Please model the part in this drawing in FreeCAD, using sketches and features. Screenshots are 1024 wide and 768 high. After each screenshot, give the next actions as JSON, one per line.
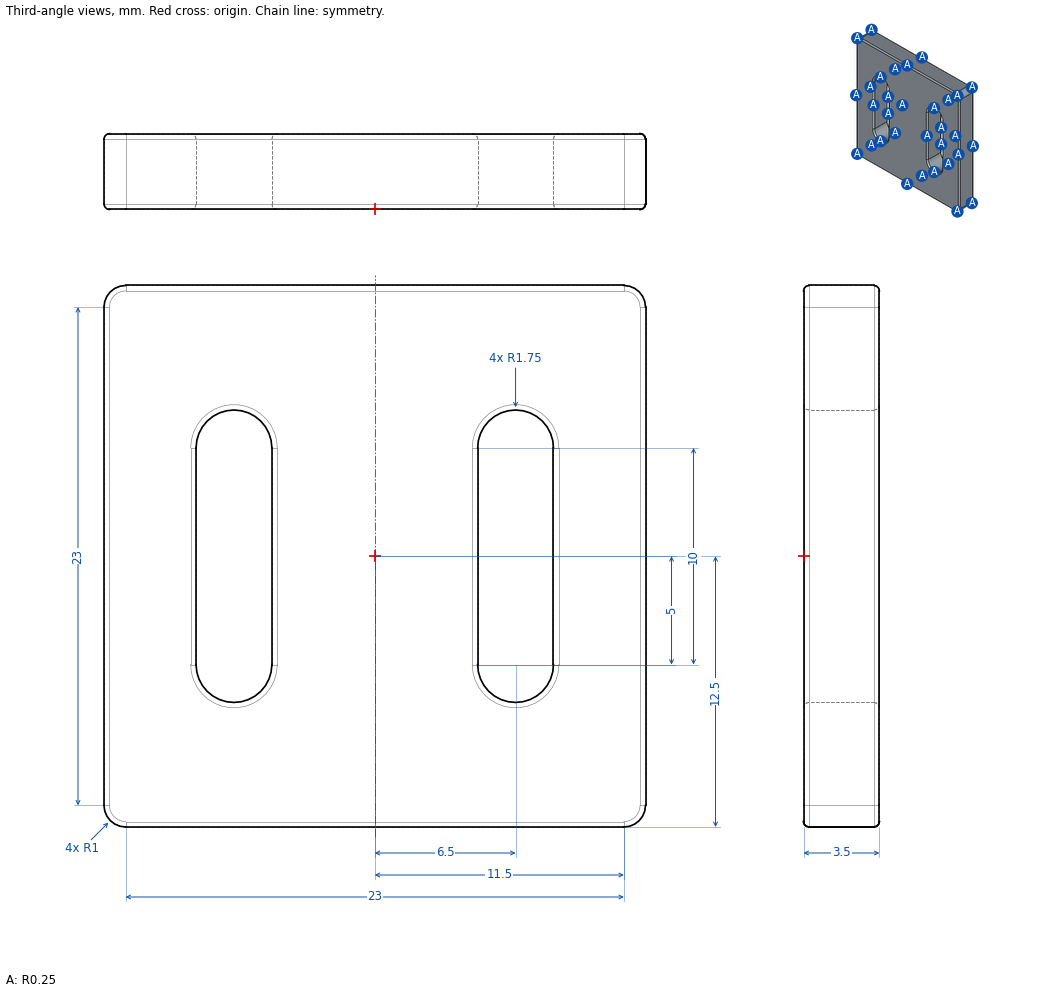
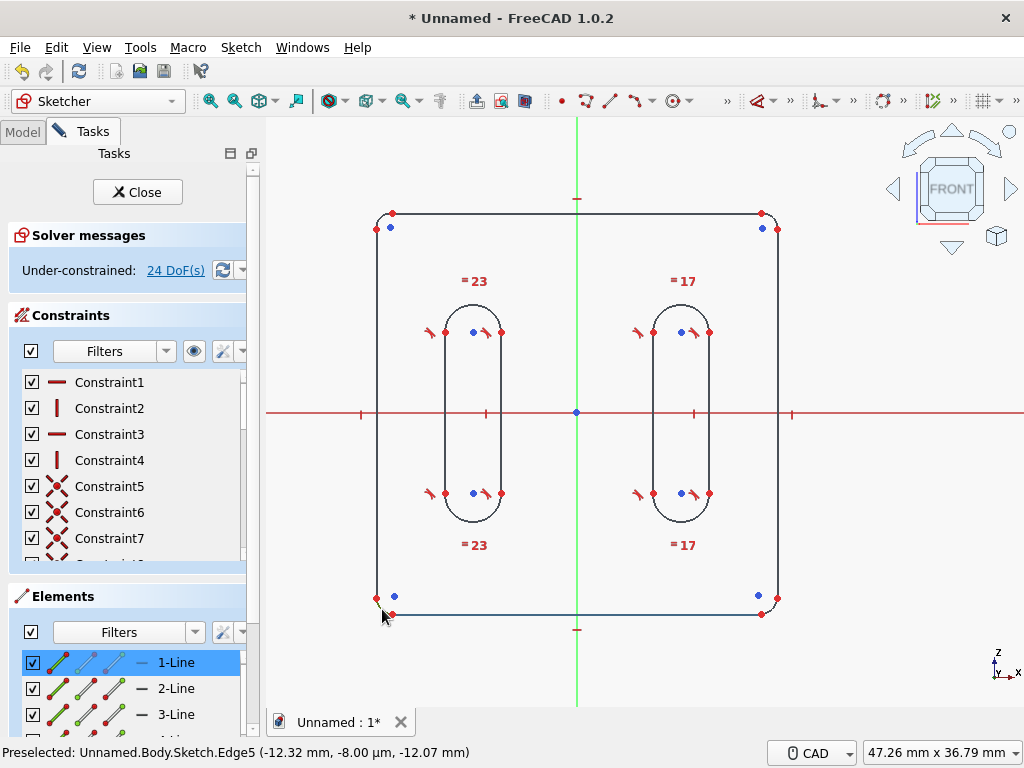
{"action": "key", "text": "t"}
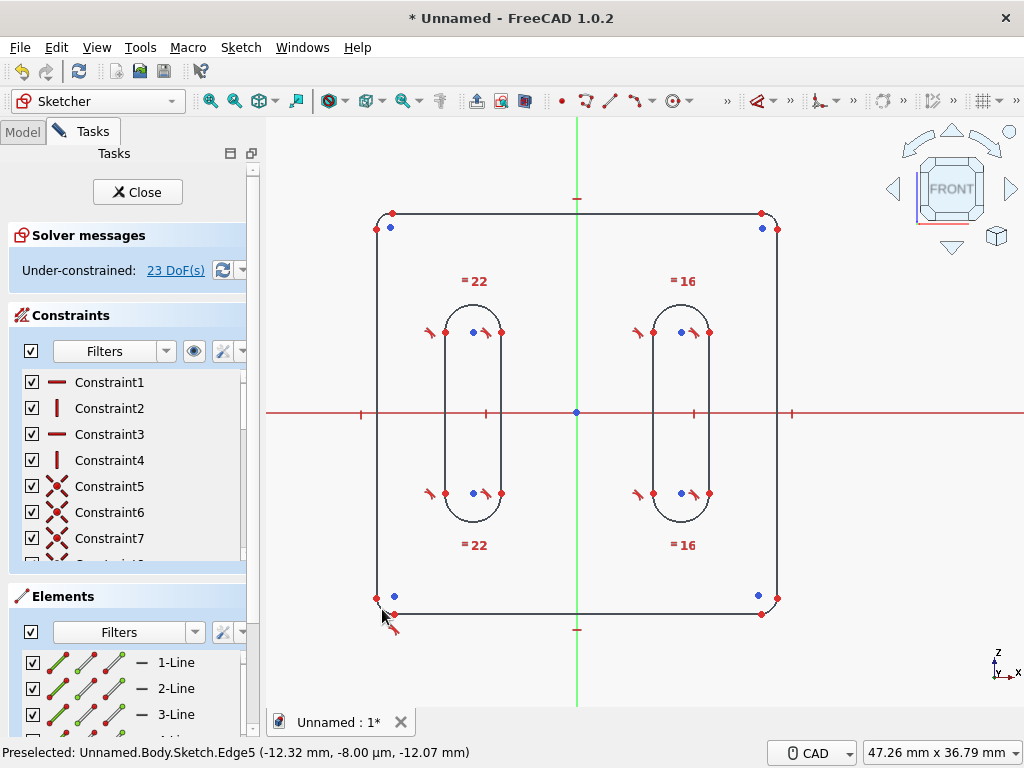
{"action": "left_click", "coordinate": [651, 614]}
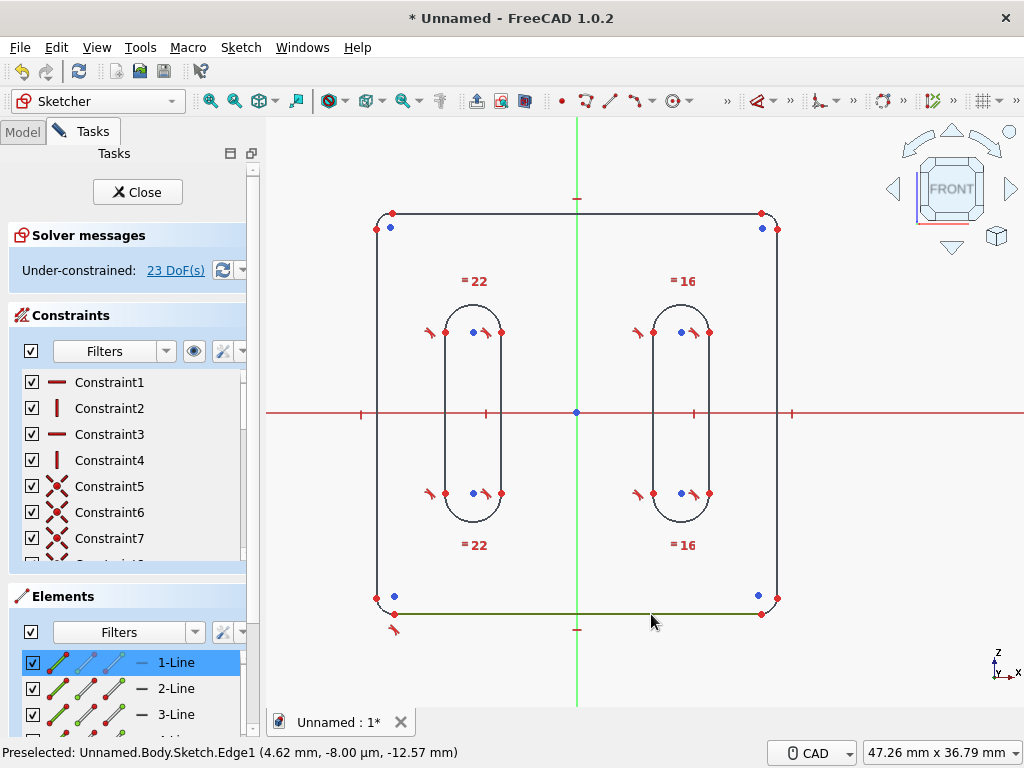
{"action": "left_click", "coordinate": [772, 609]}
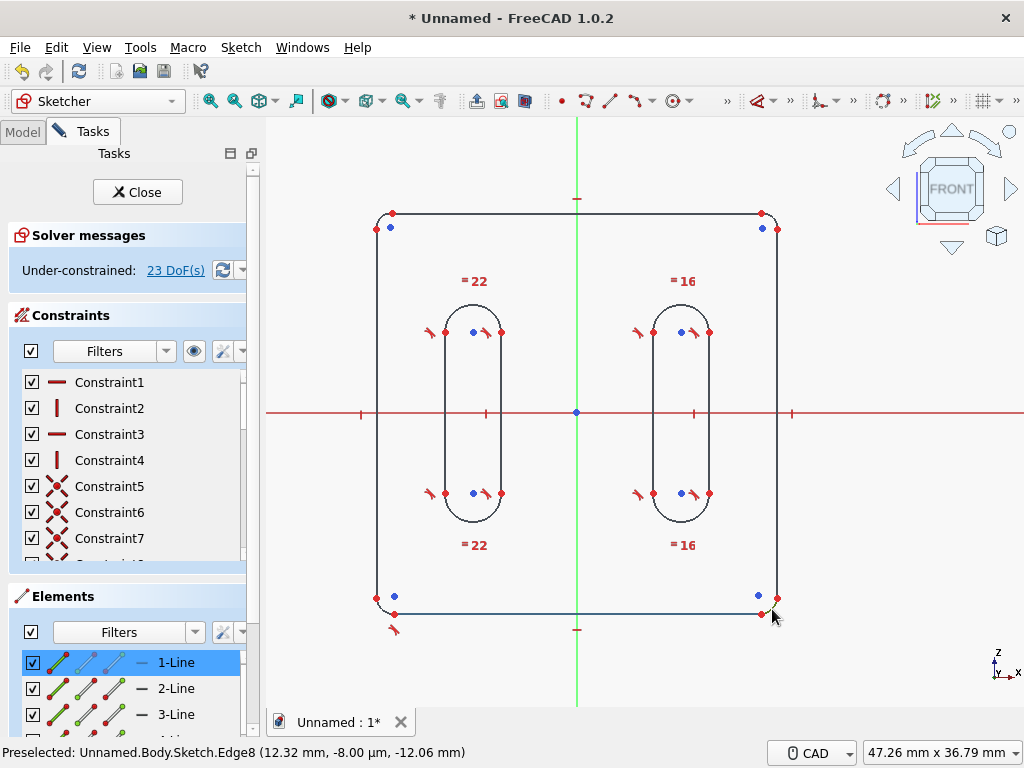
{"action": "key", "text": "t"}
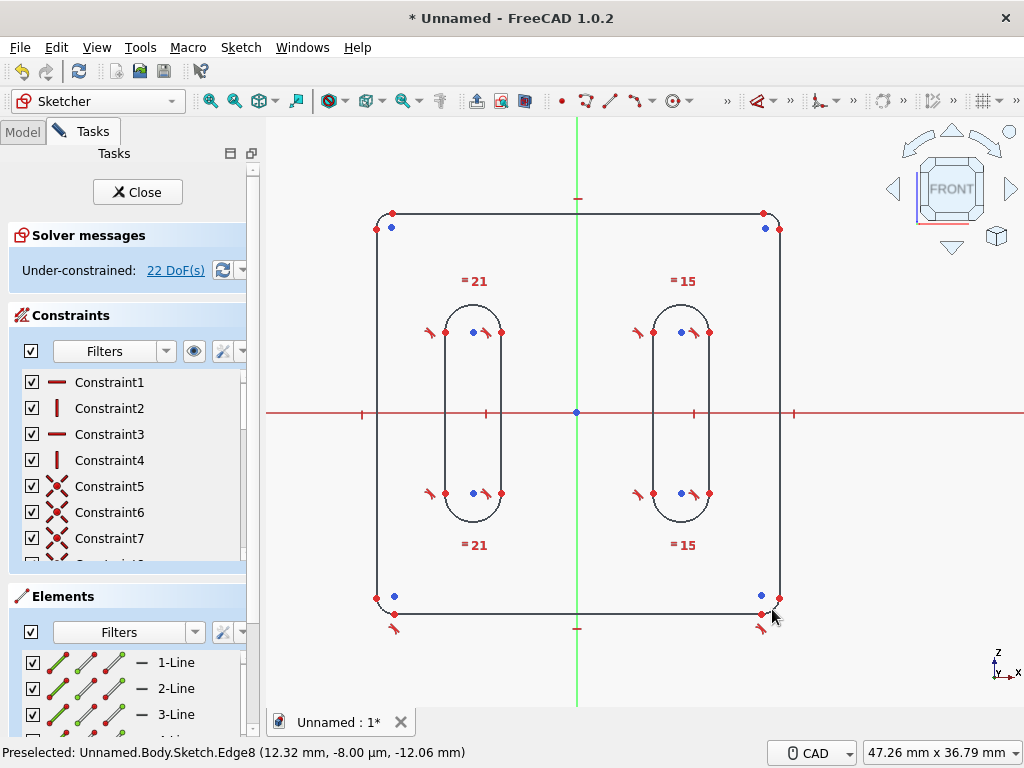
{"action": "left_click", "coordinate": [377, 488]}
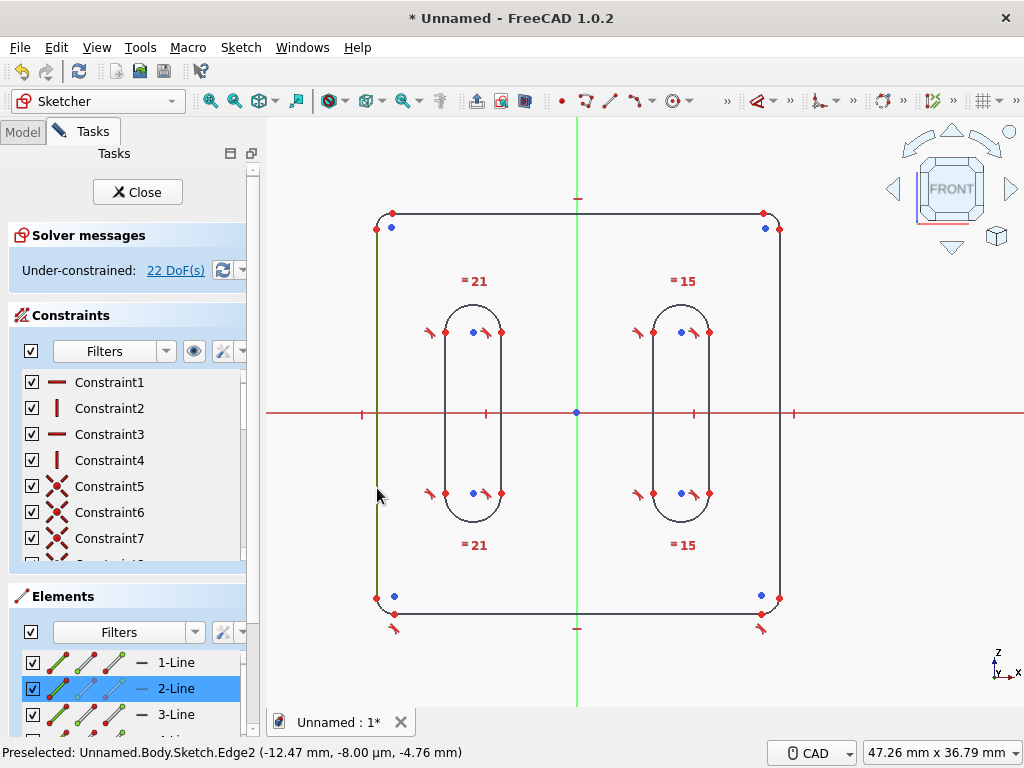
{"action": "left_click", "coordinate": [383, 610]}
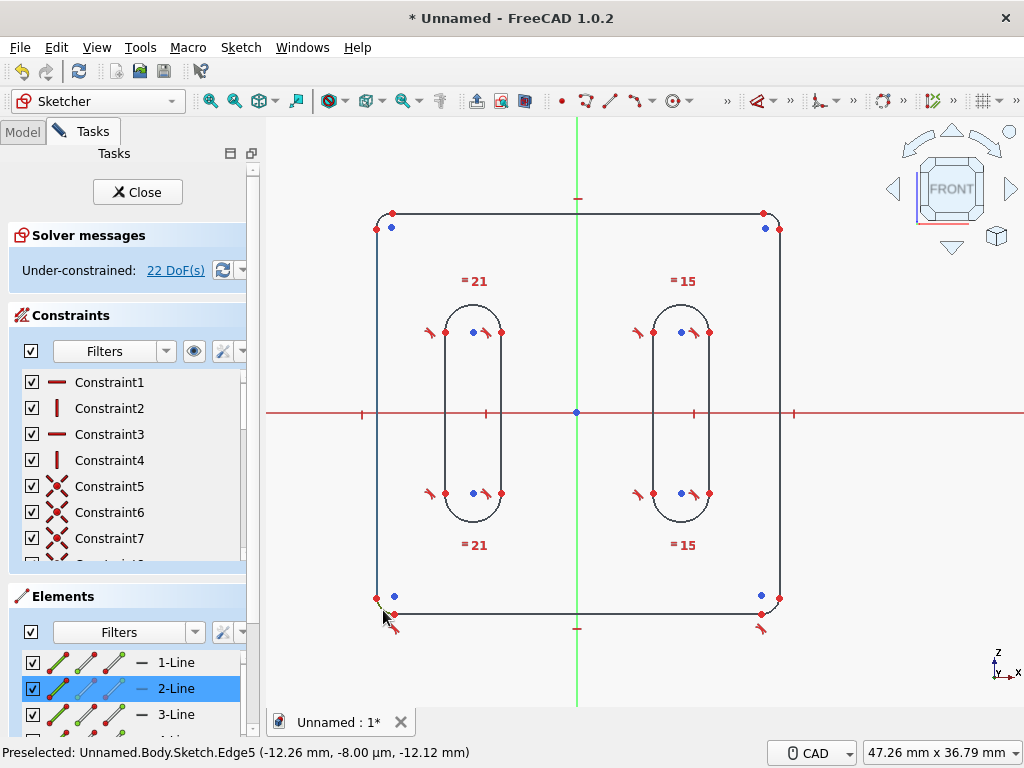
{"action": "key", "text": "t"}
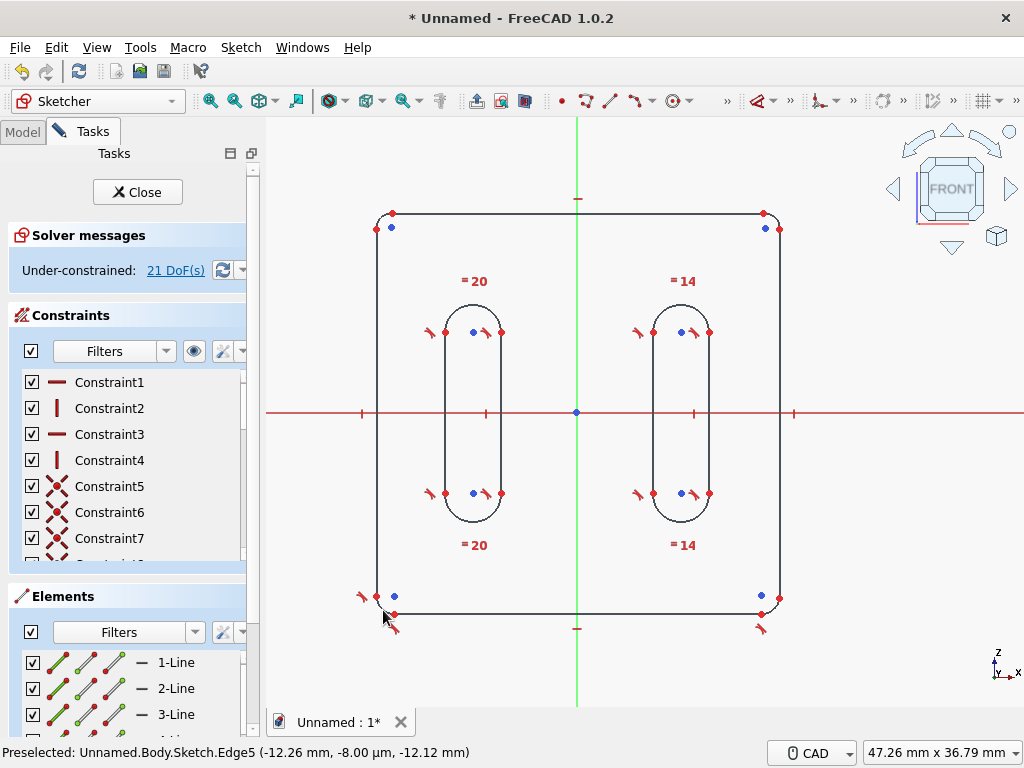
{"action": "left_click", "coordinate": [377, 486]}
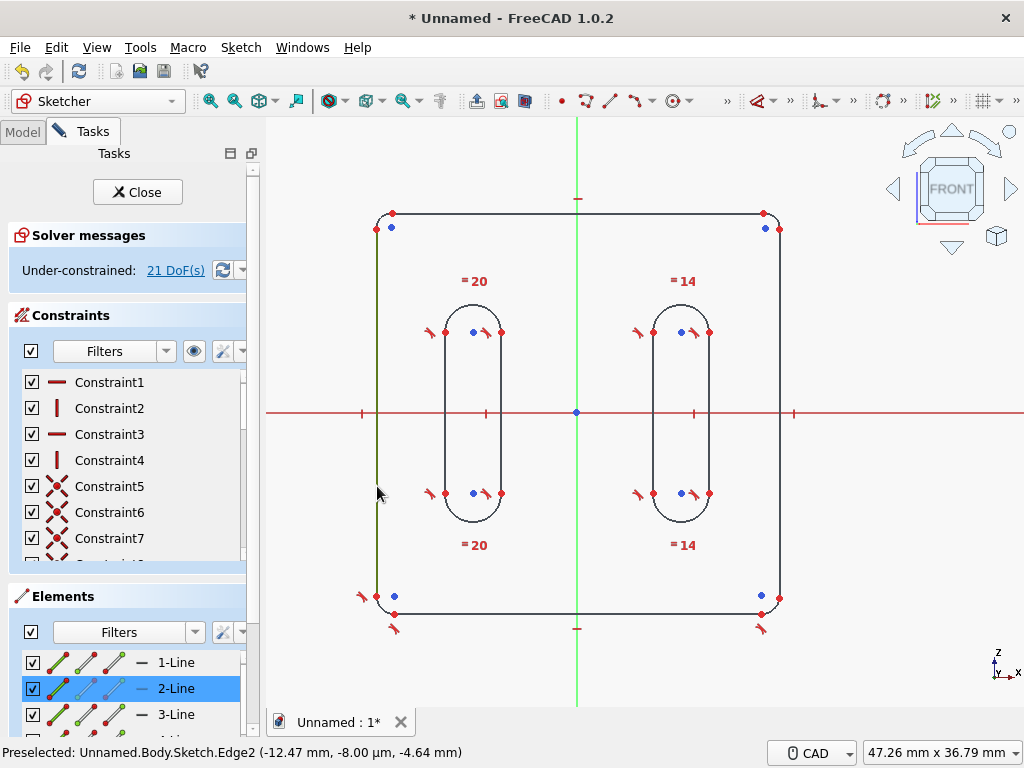
{"action": "left_click", "coordinate": [381, 218]}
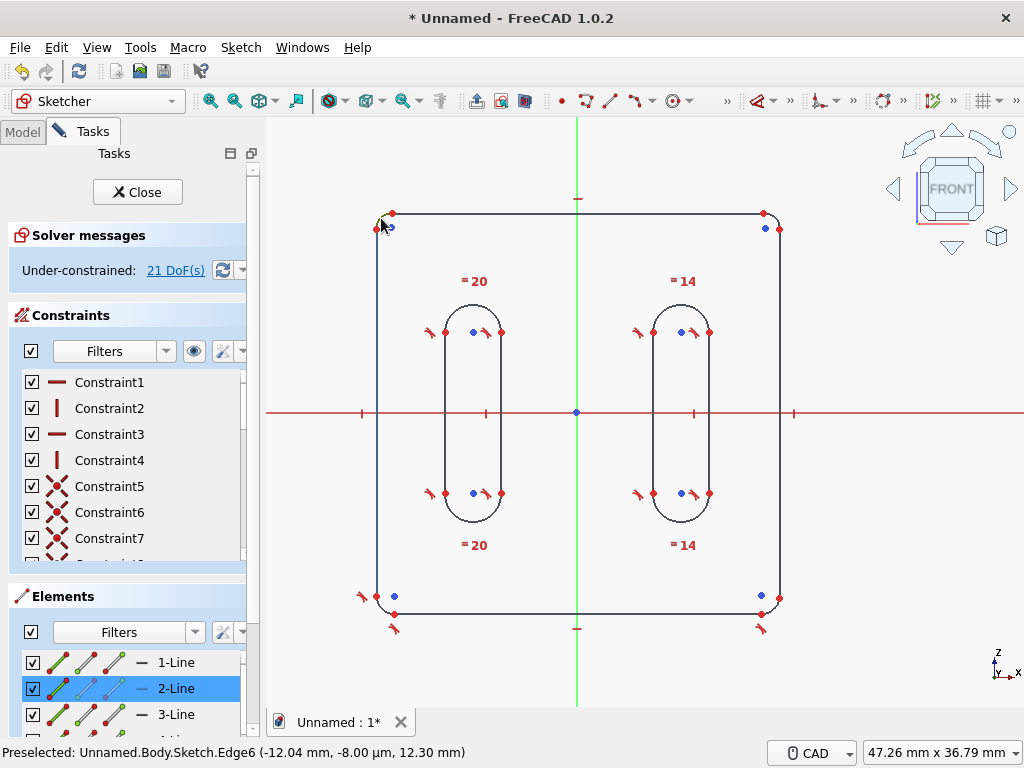
{"action": "key", "text": "t"}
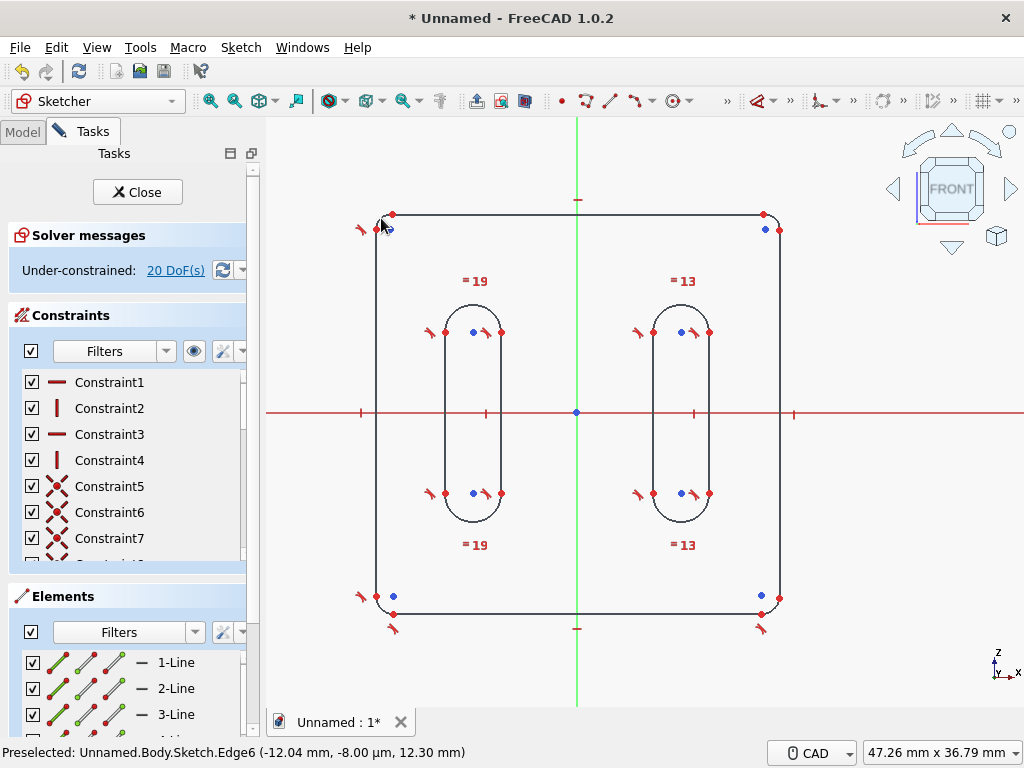
{"action": "left_click", "coordinate": [504, 215]}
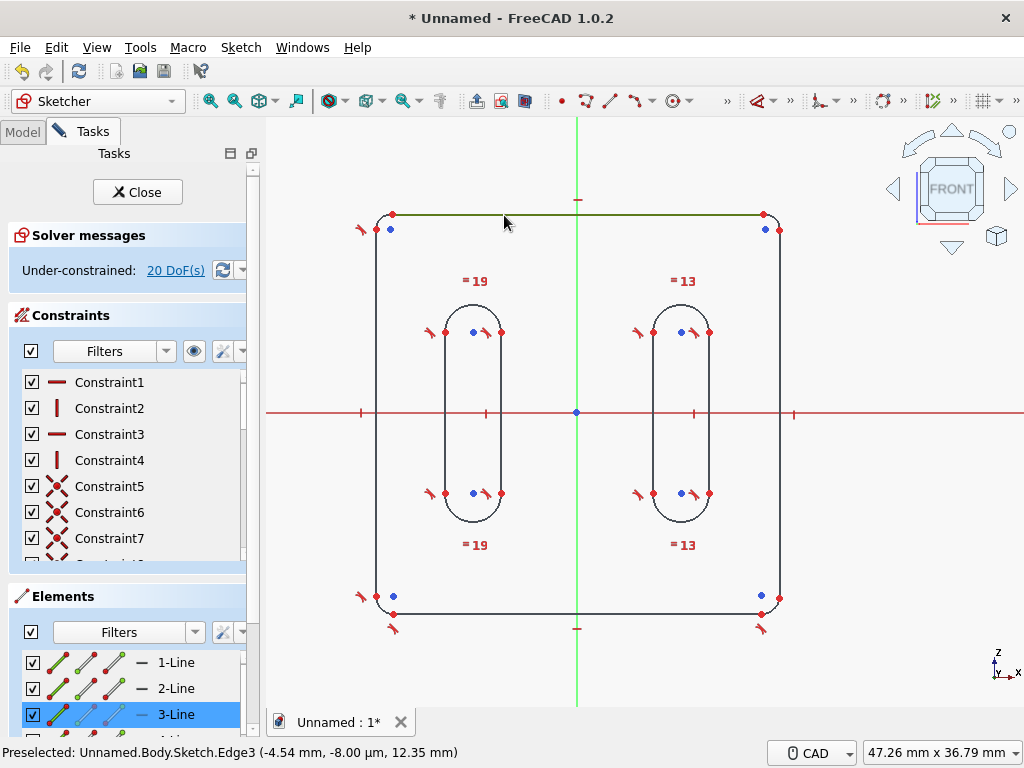
{"action": "left_click", "coordinate": [381, 218]}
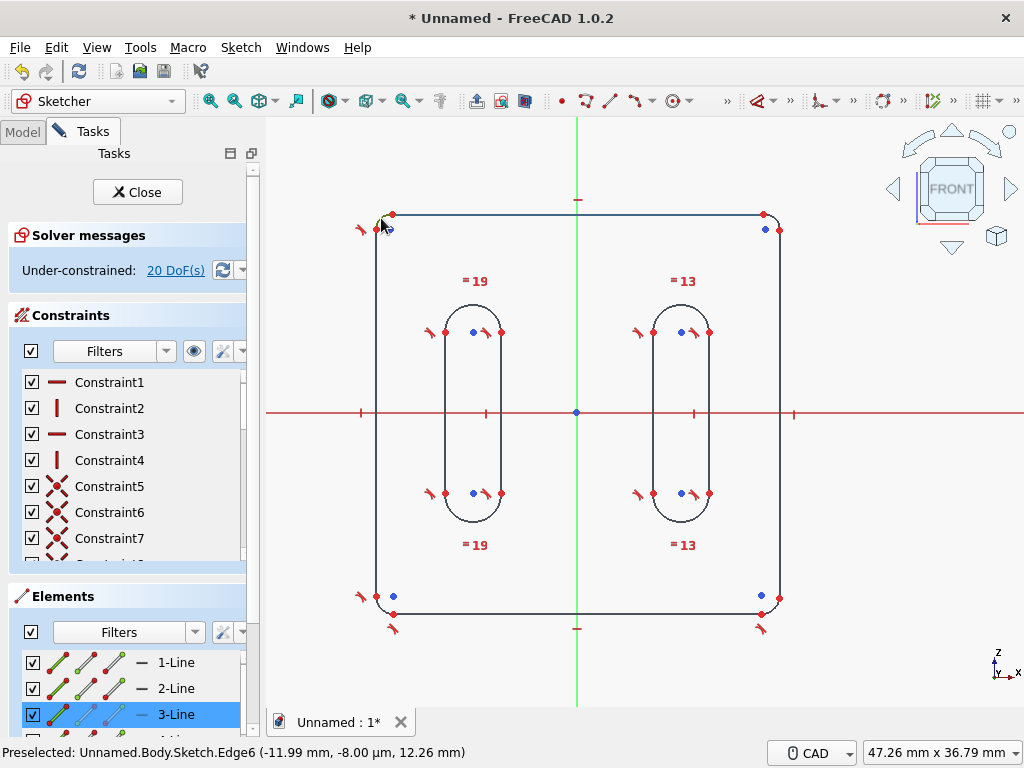
{"action": "key", "text": "t"}